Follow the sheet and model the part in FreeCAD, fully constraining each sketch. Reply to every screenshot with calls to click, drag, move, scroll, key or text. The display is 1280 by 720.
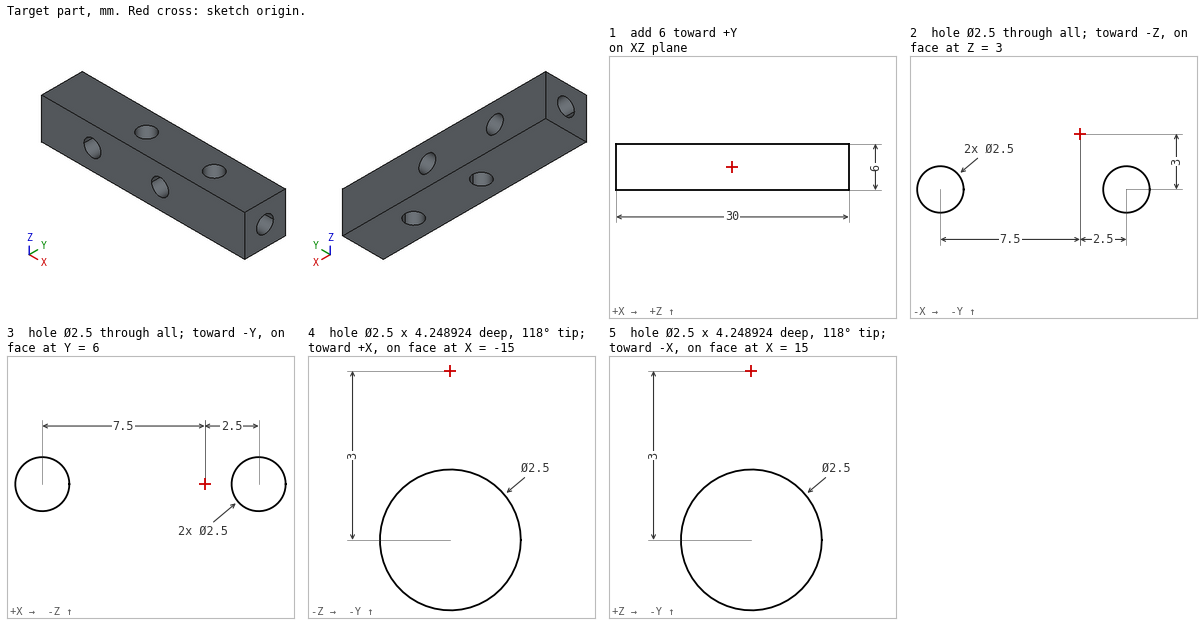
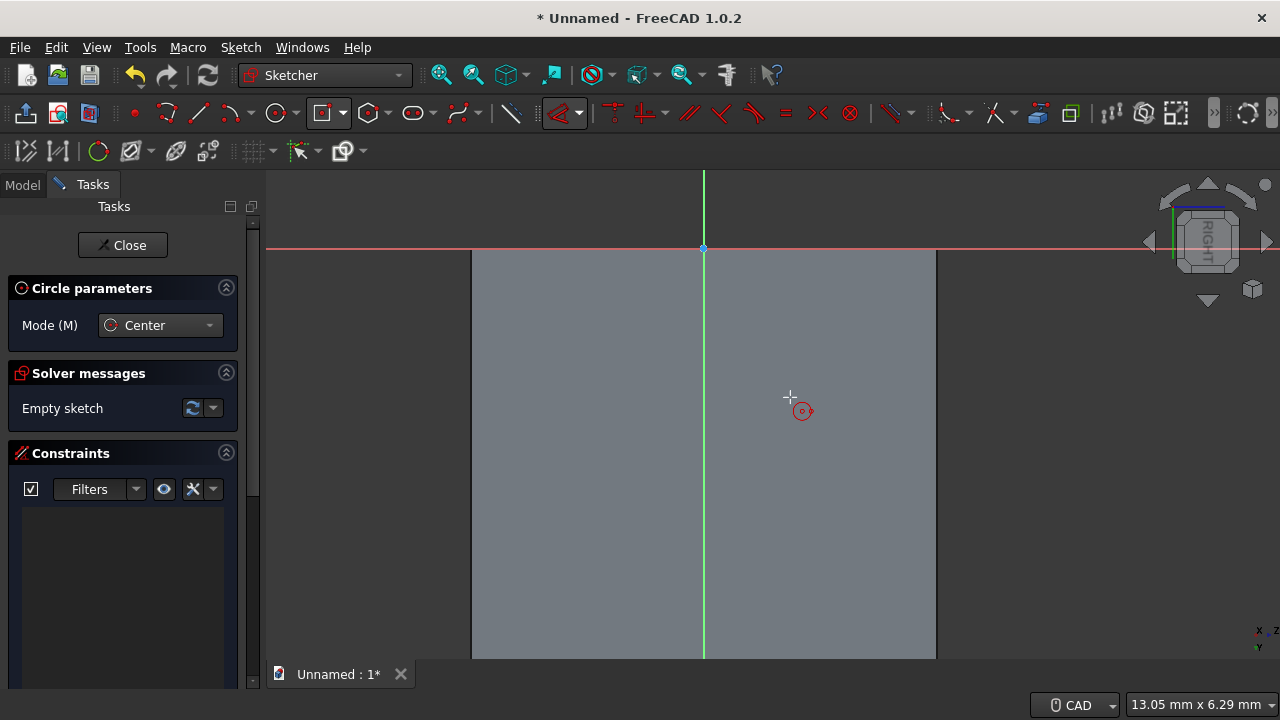
click(704, 482)
move(772, 413)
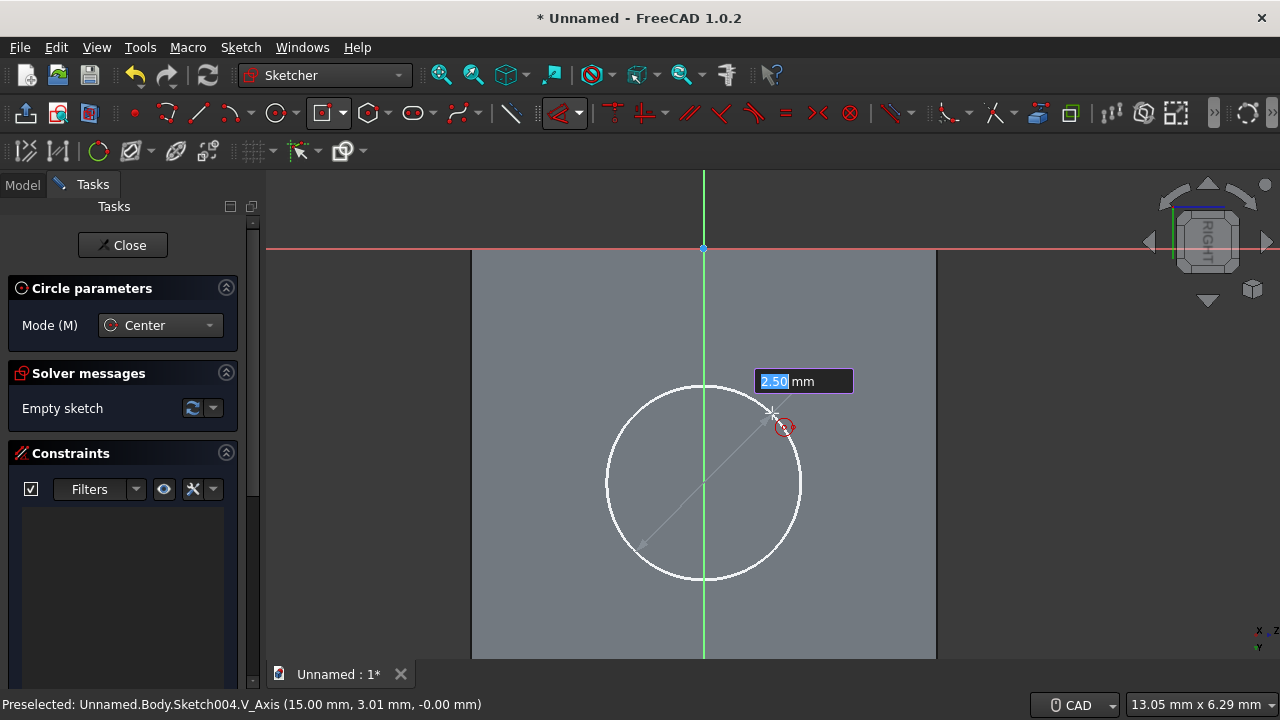
text(2.5)
key(Return)
key(Escape)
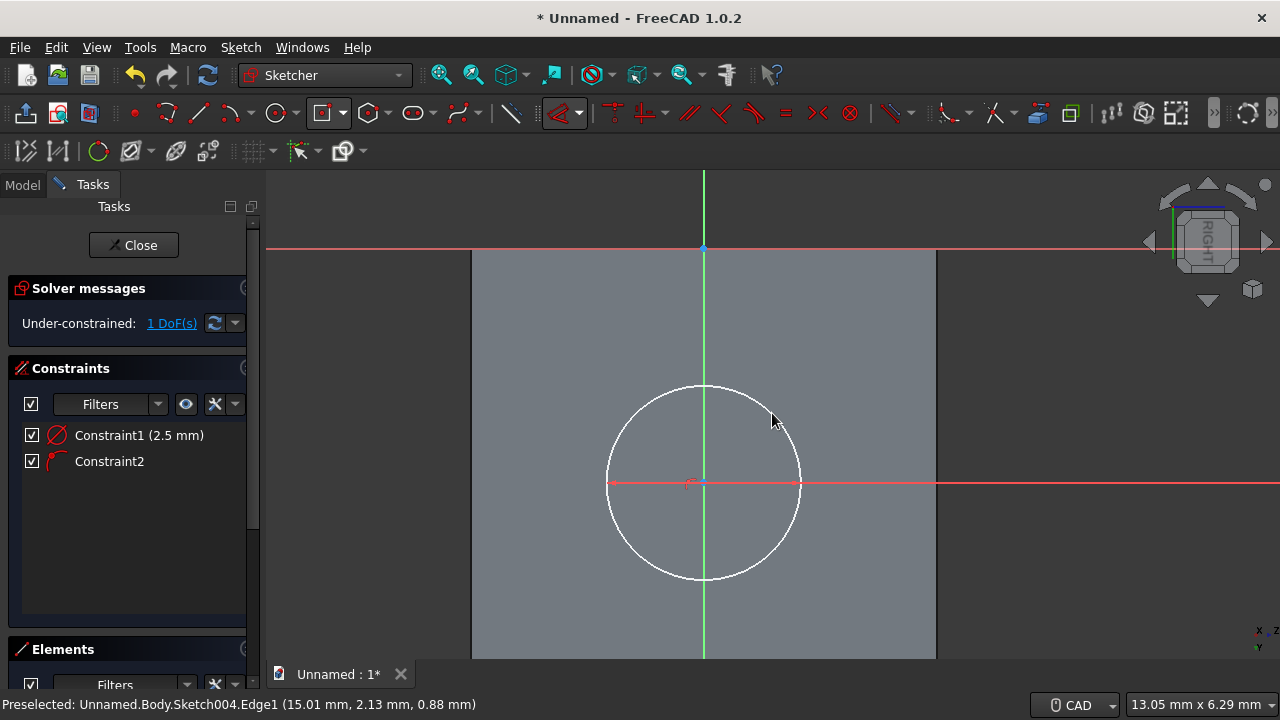
click(706, 485)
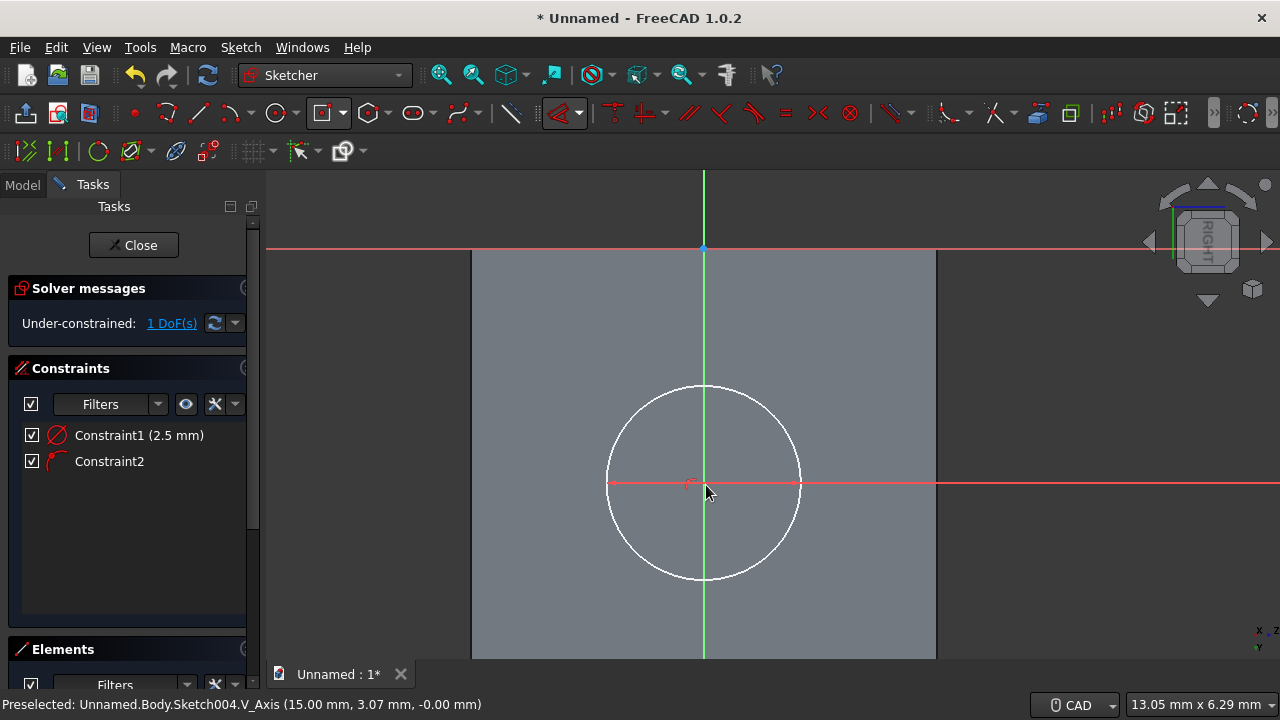
click(582, 114)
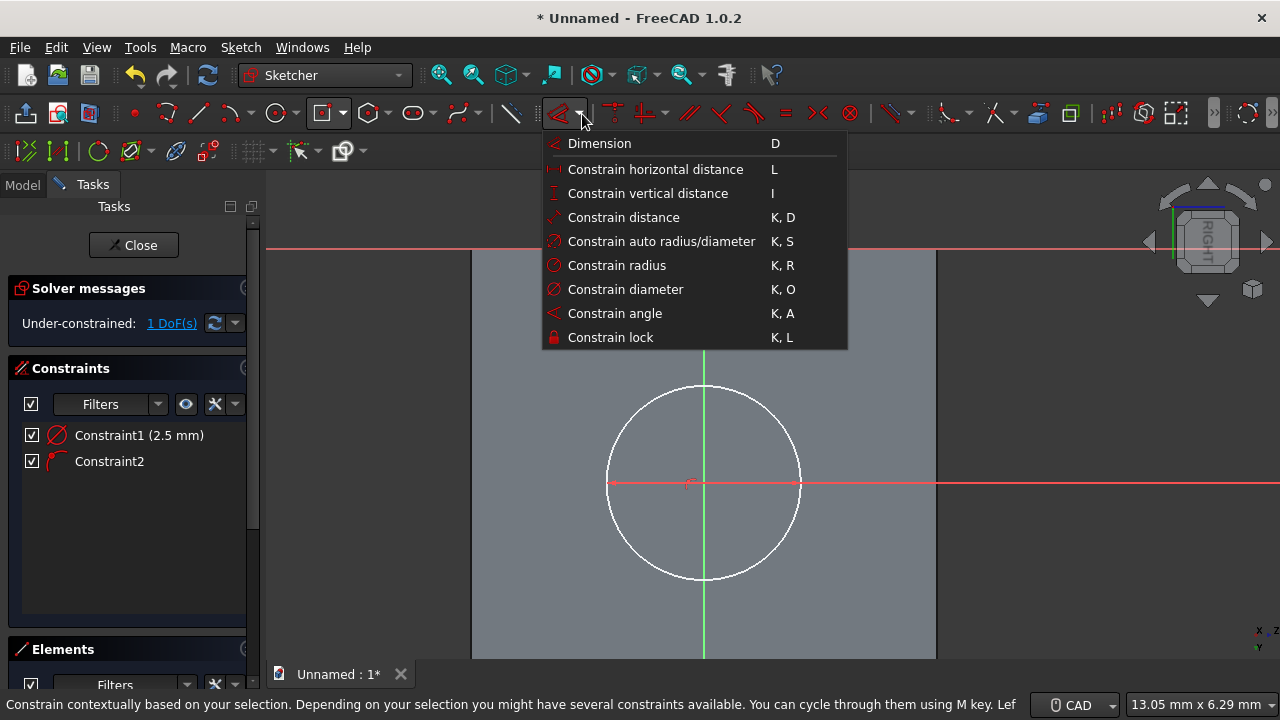
click(695, 193)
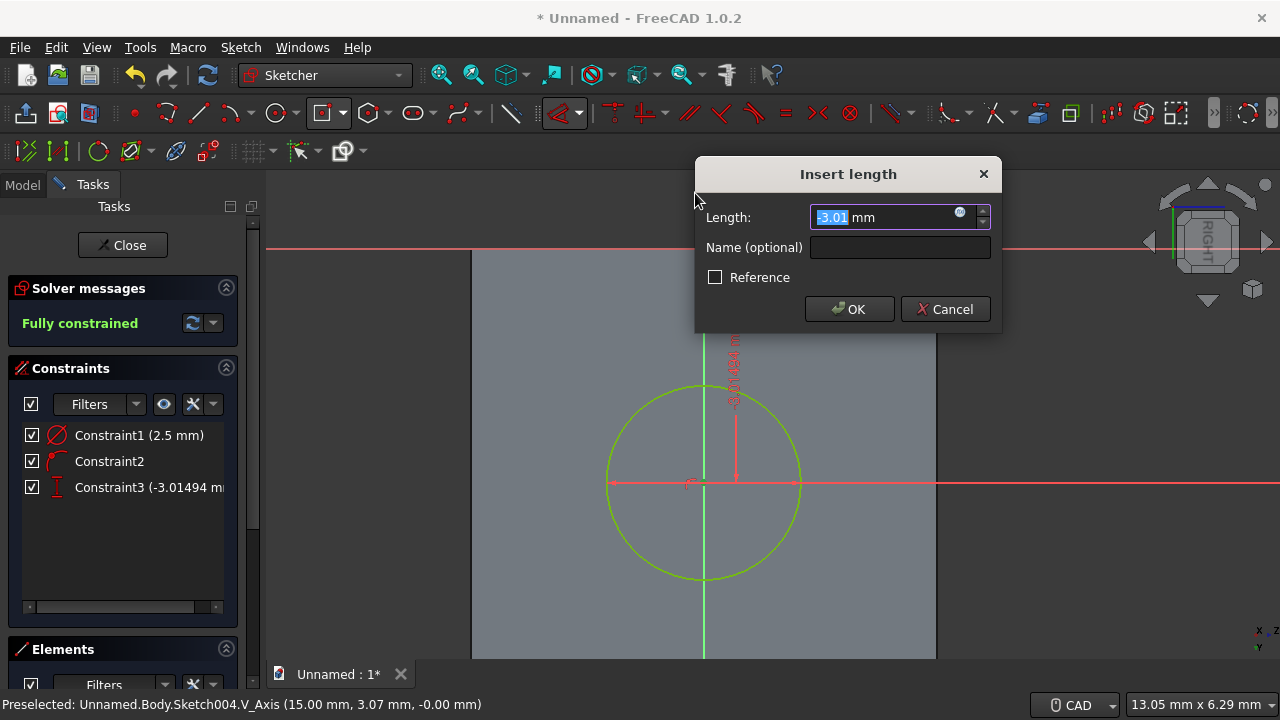
text(-3)
key(Return)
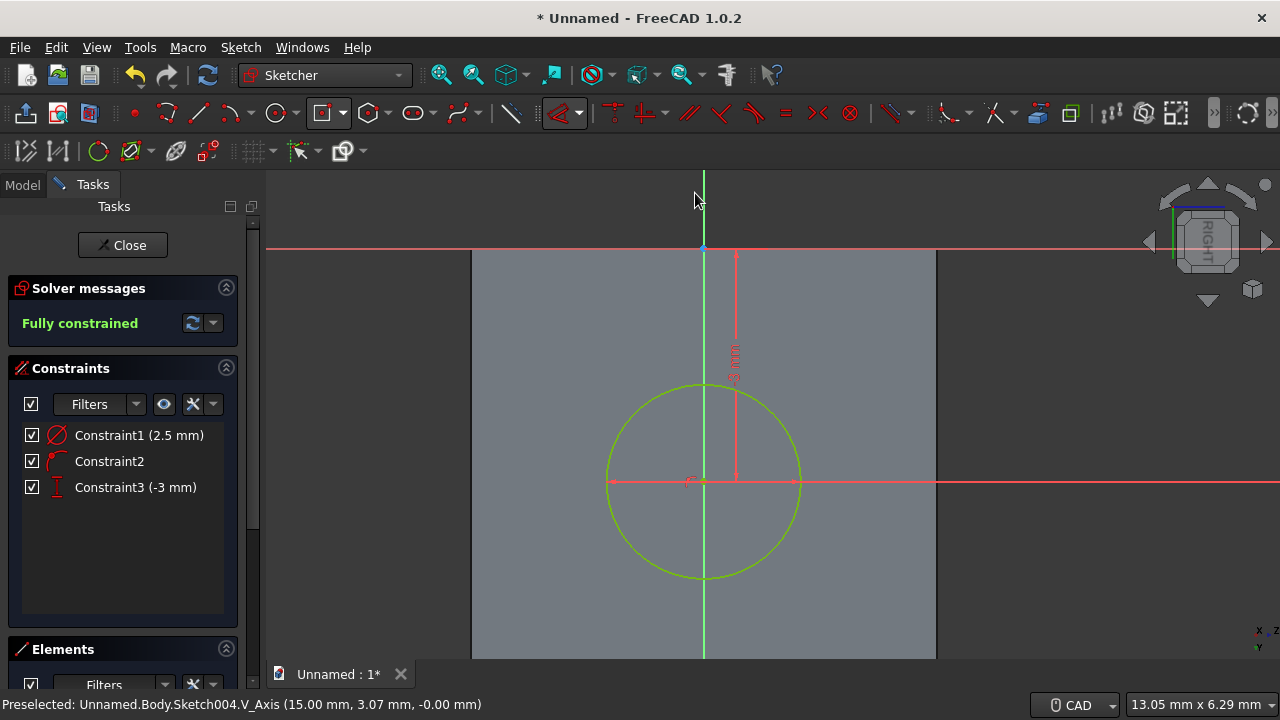
click(123, 245)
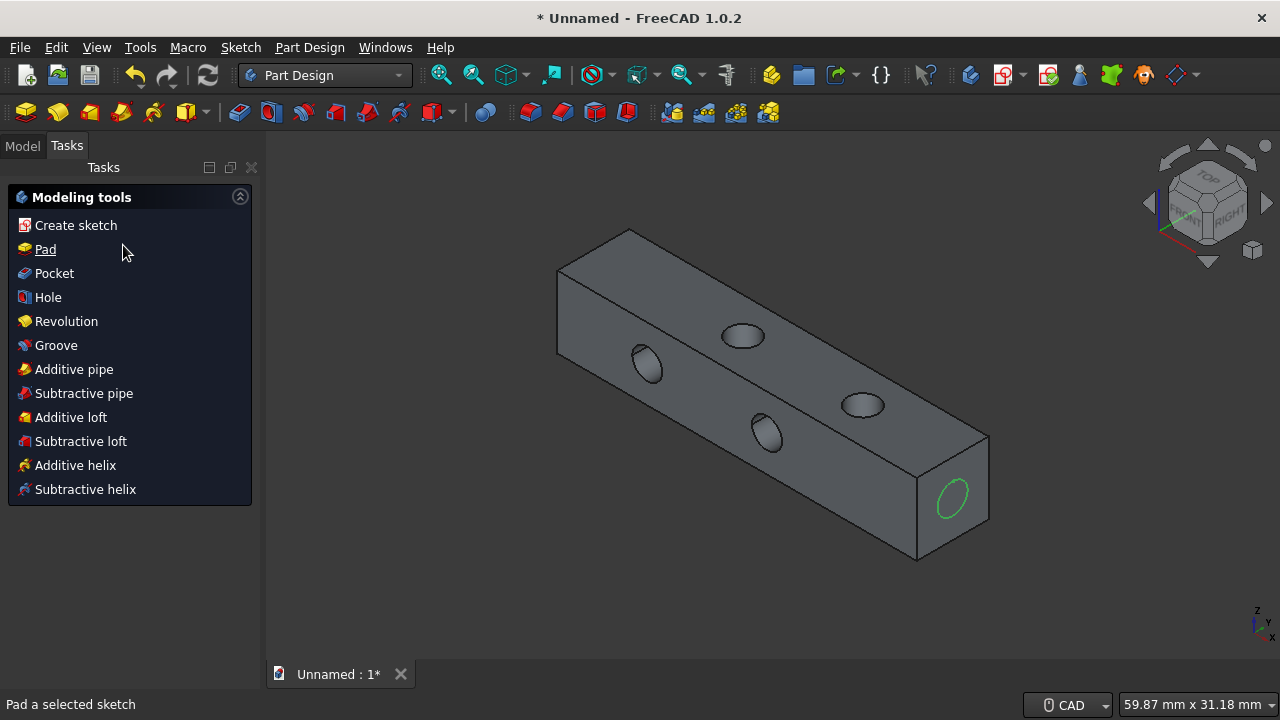
click(272, 112)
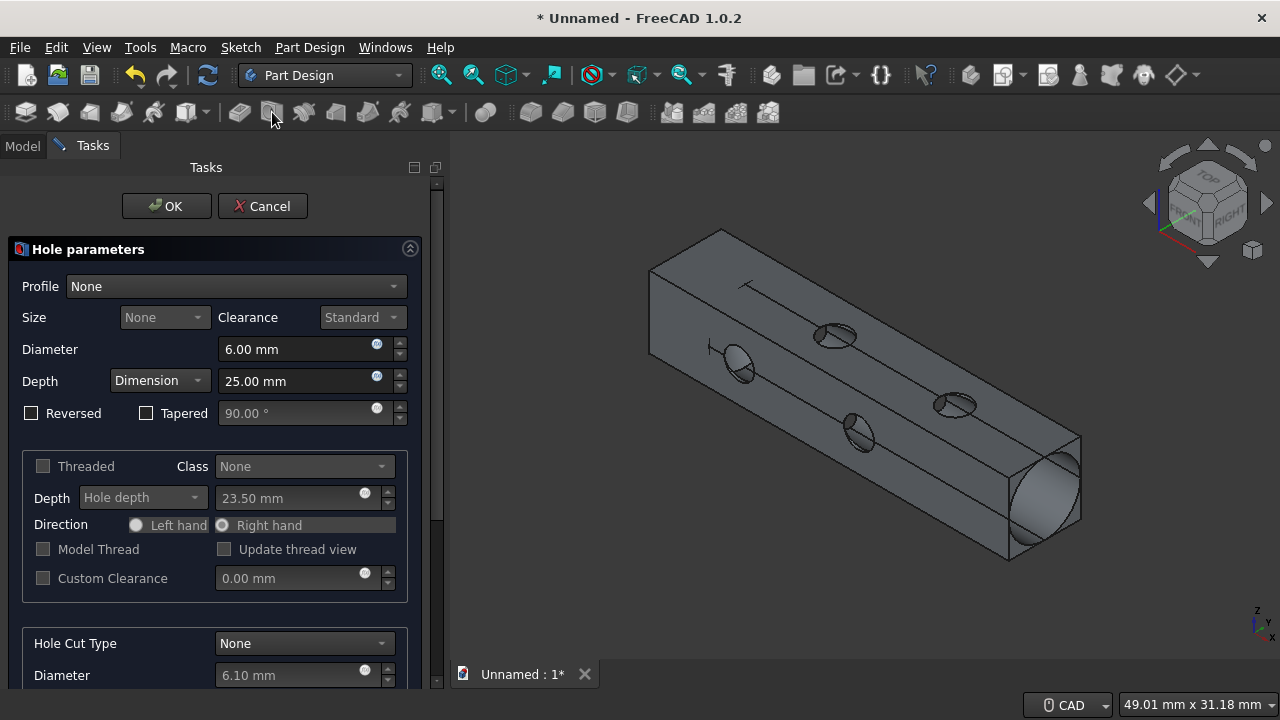
triple_click(305, 349)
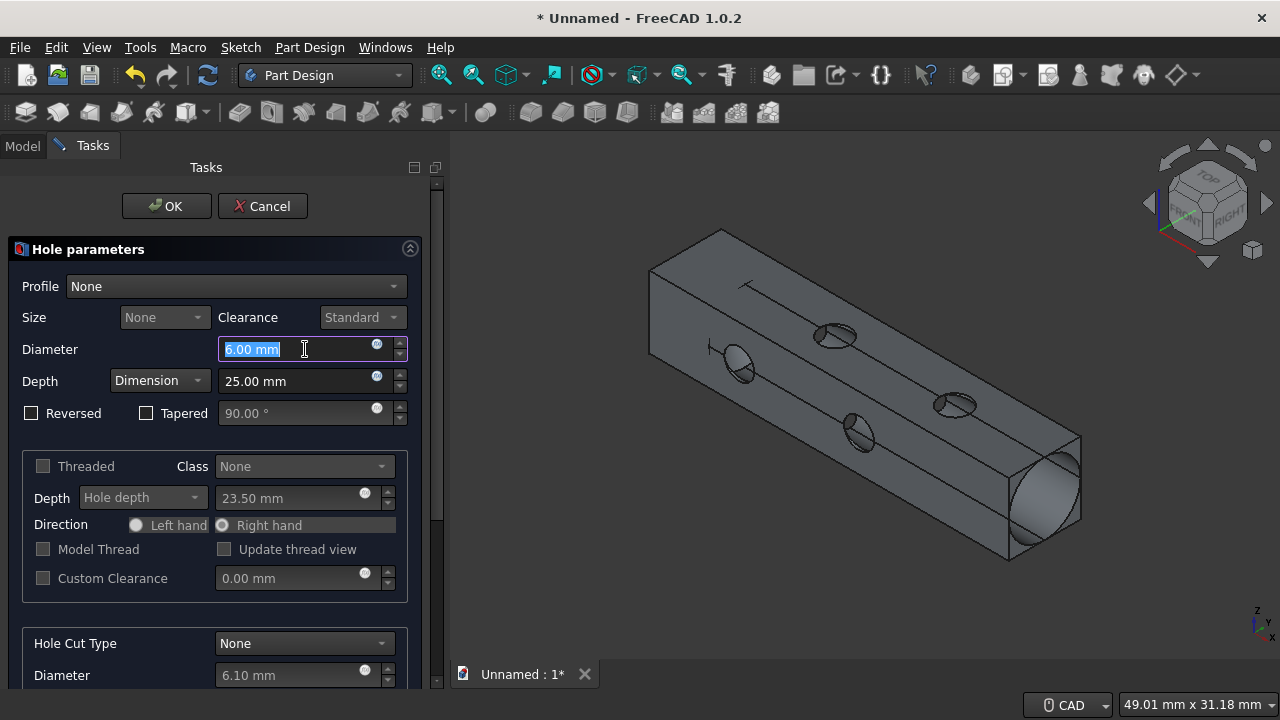
text(2.5)
key(Tab)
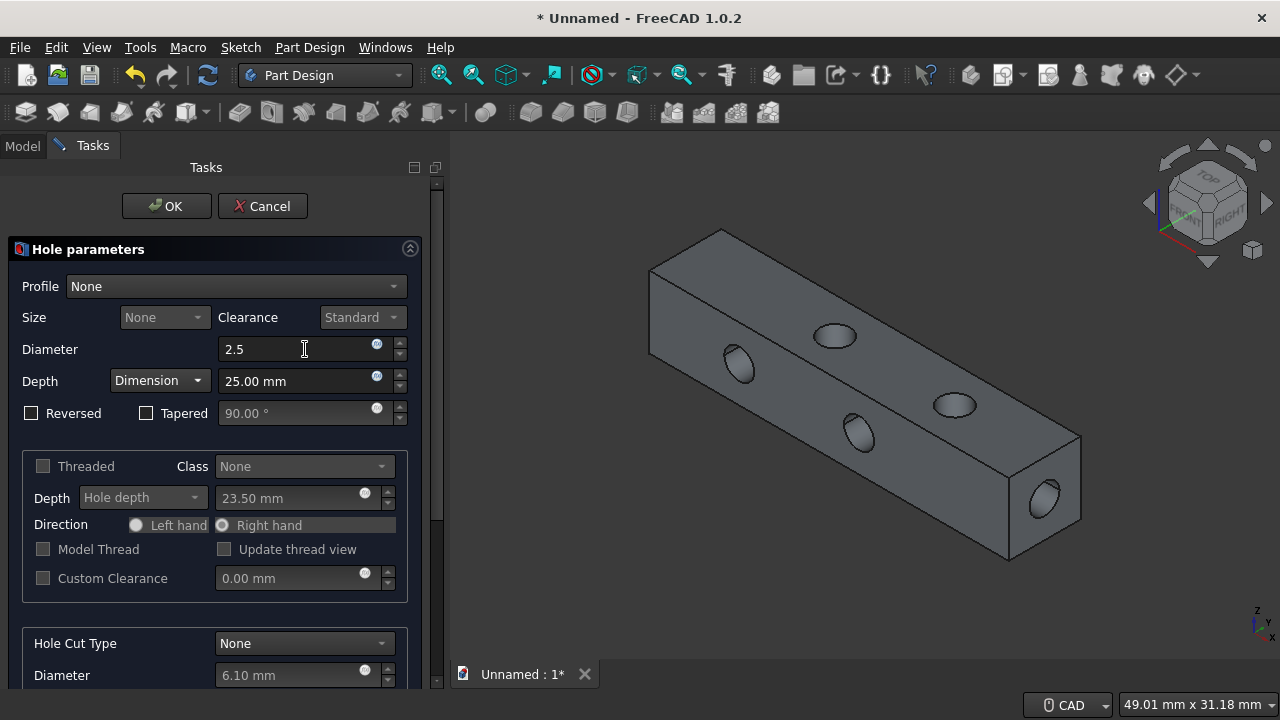
triple_click(305, 381)